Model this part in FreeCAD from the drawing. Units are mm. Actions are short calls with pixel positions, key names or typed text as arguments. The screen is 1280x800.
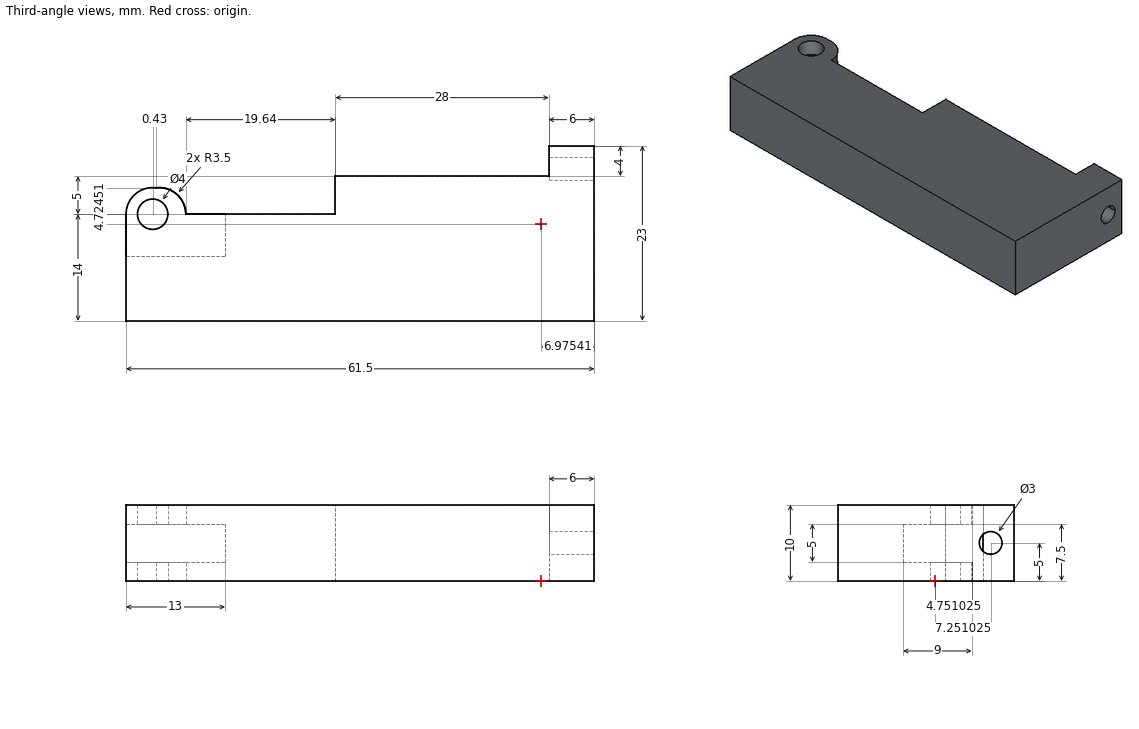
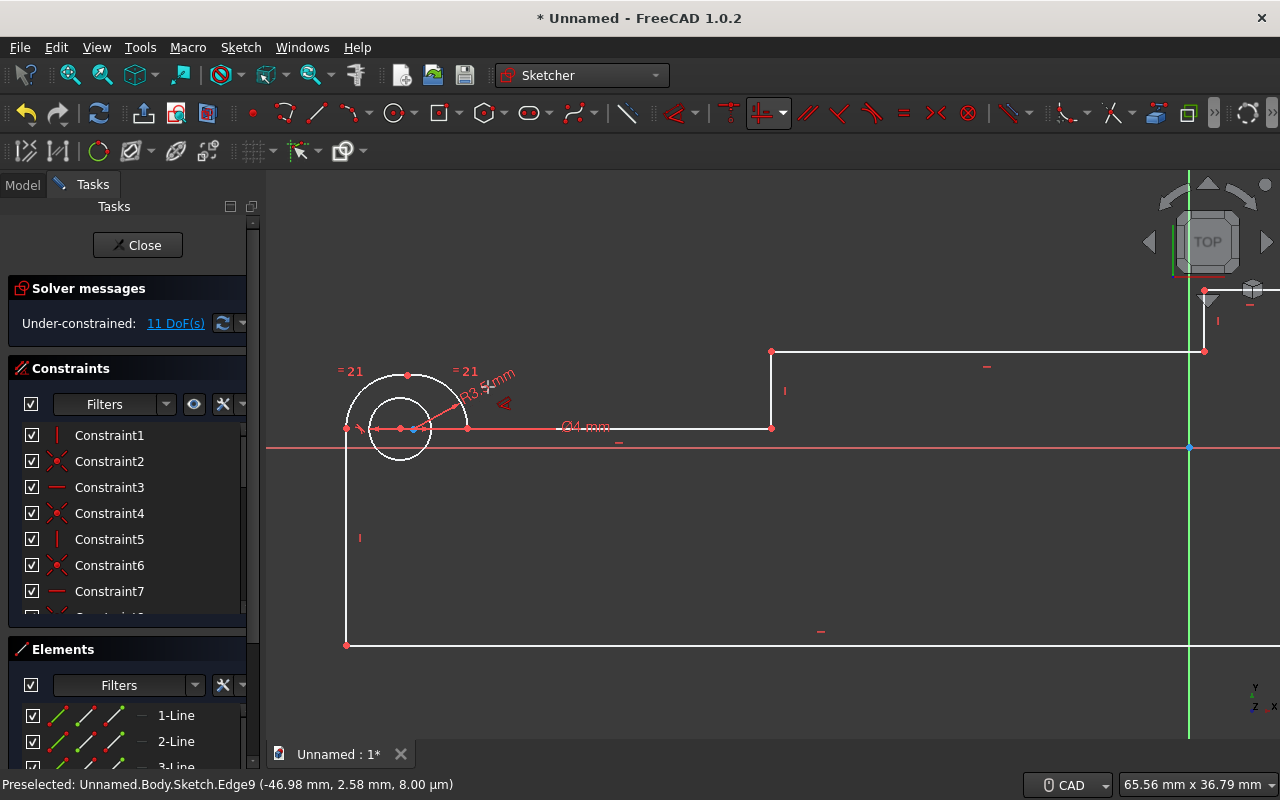
scroll(467, 429, down, 2)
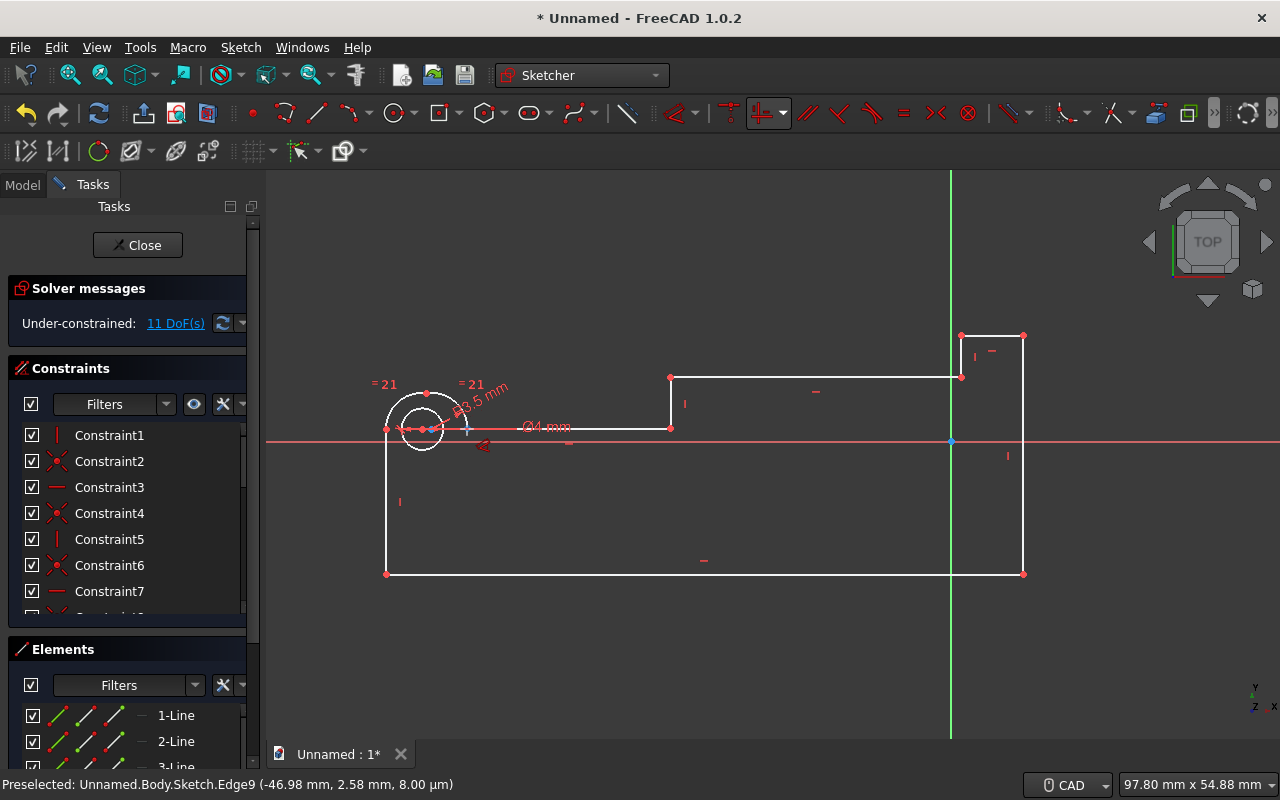
click(1004, 336)
click(992, 302)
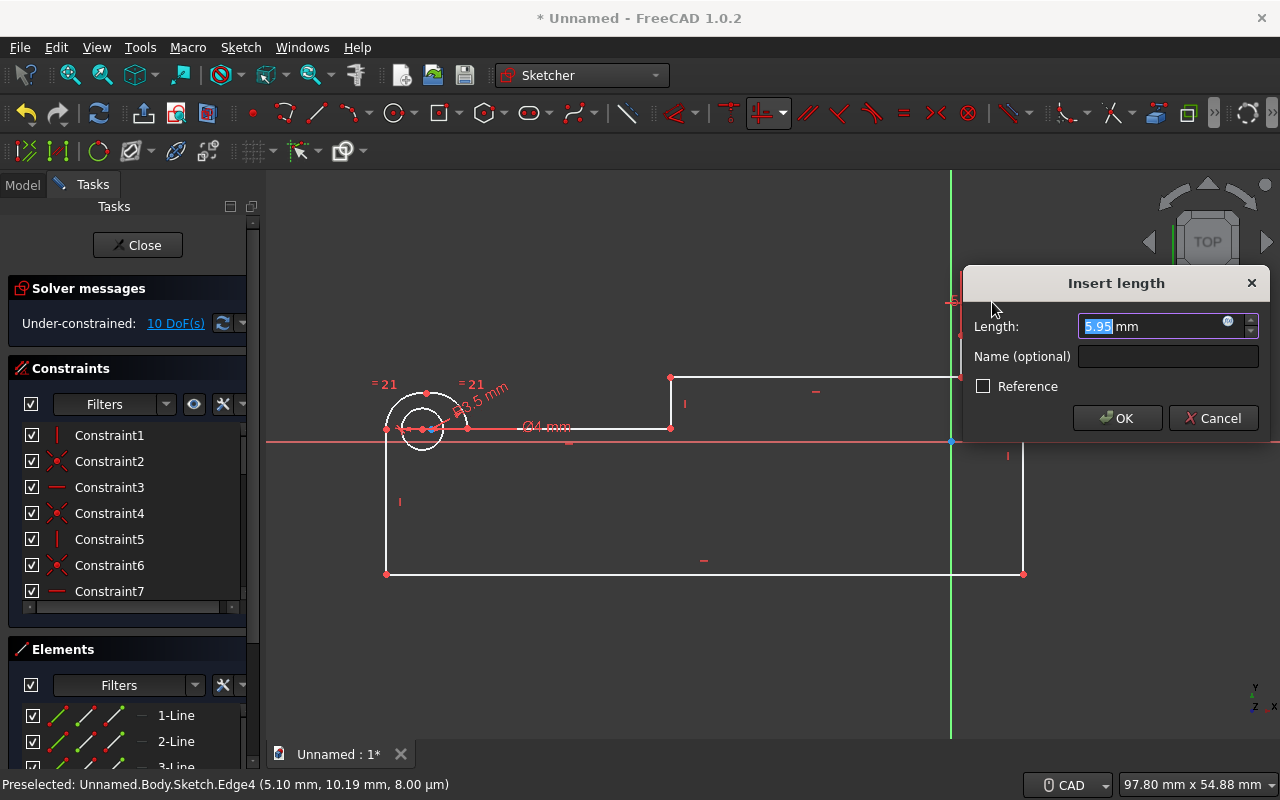
text(6)
key(Return)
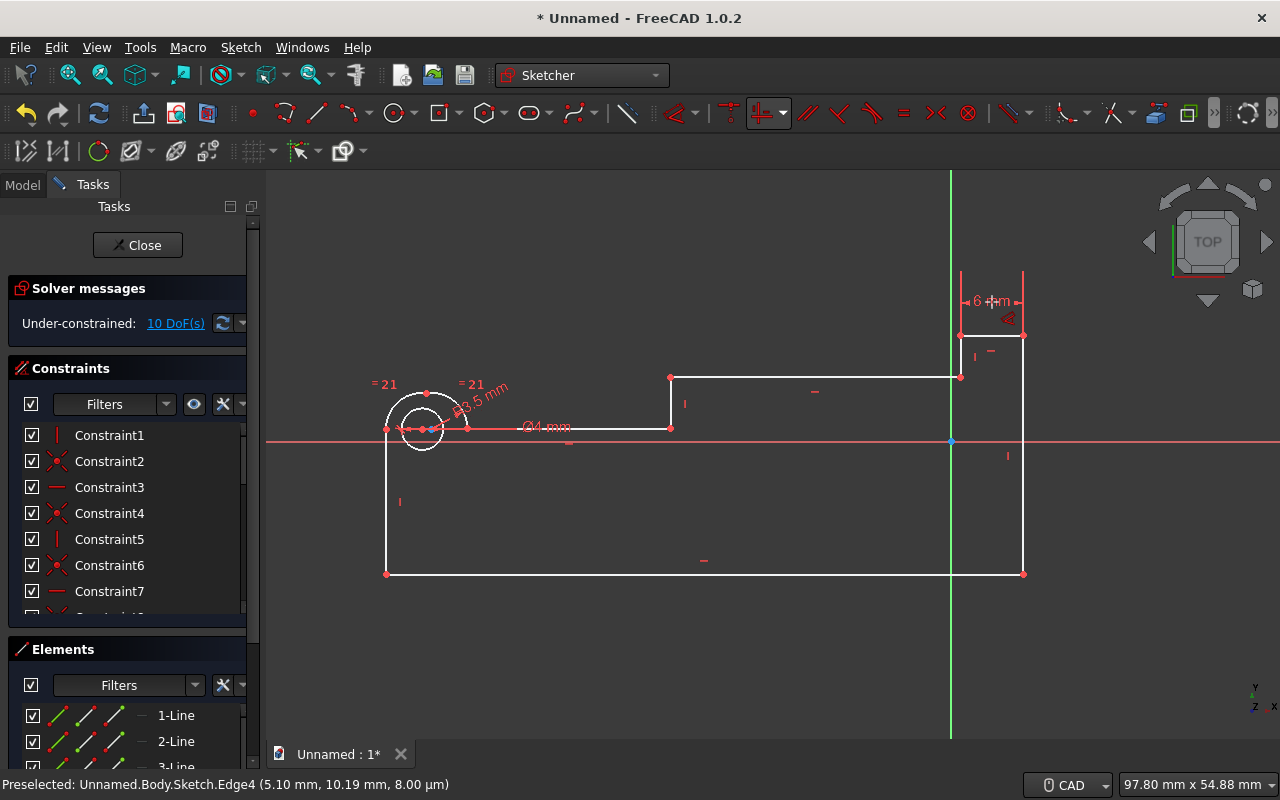
scroll(961, 348, up, 2)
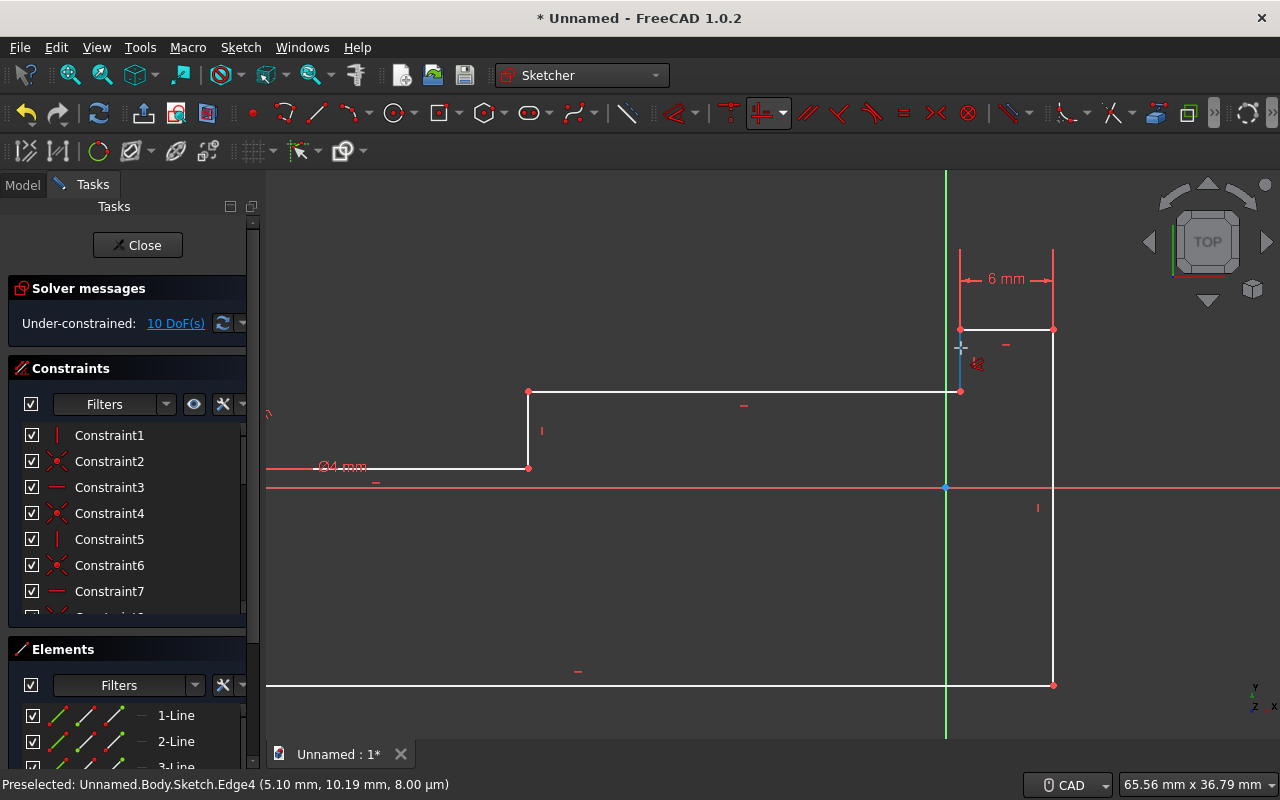
click(960, 348)
click(994, 361)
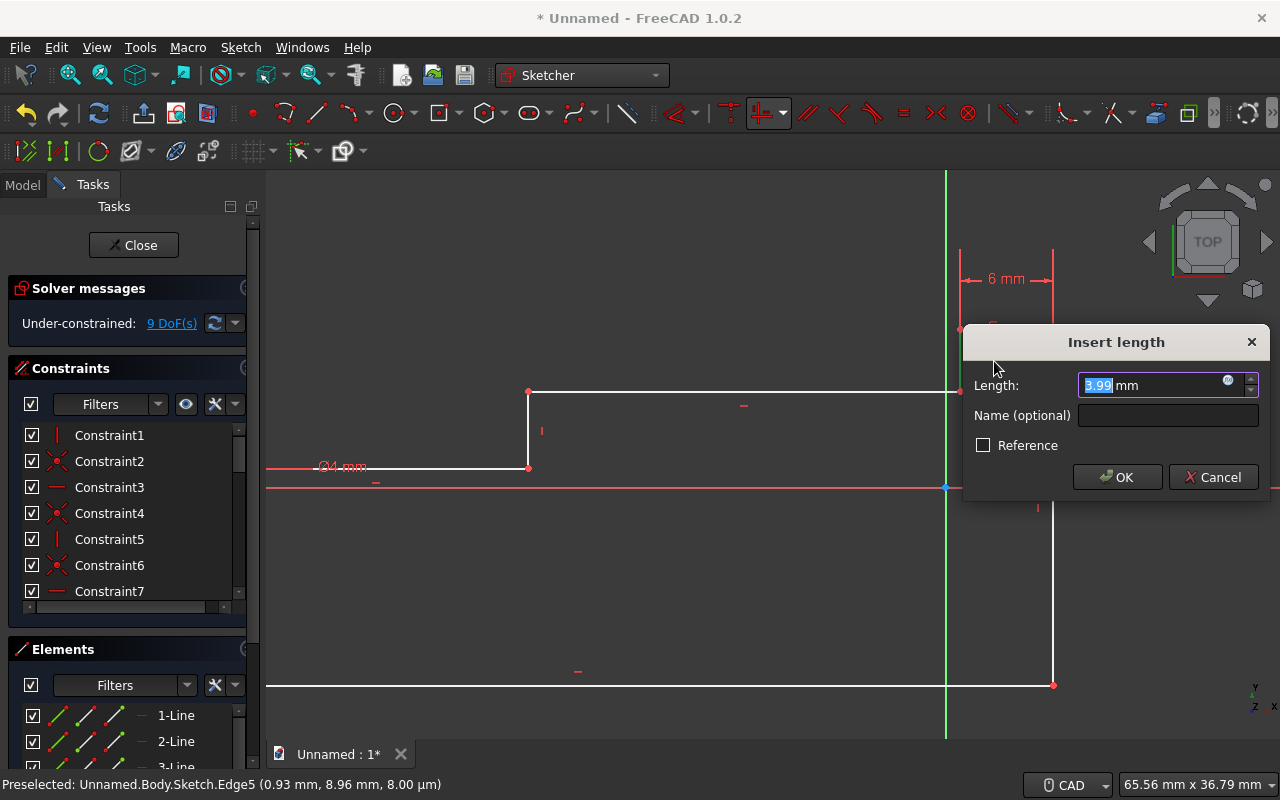
text(4)
key(Return)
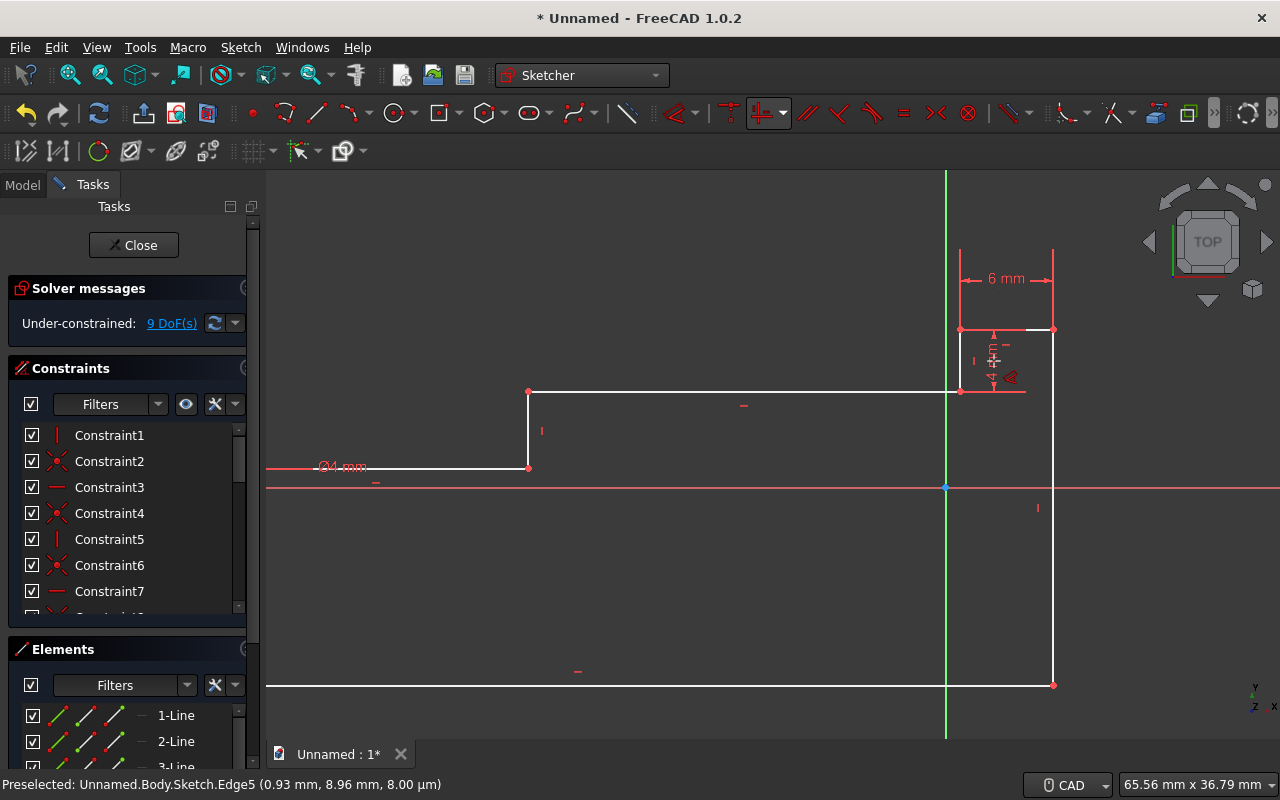
click(528, 415)
click(494, 430)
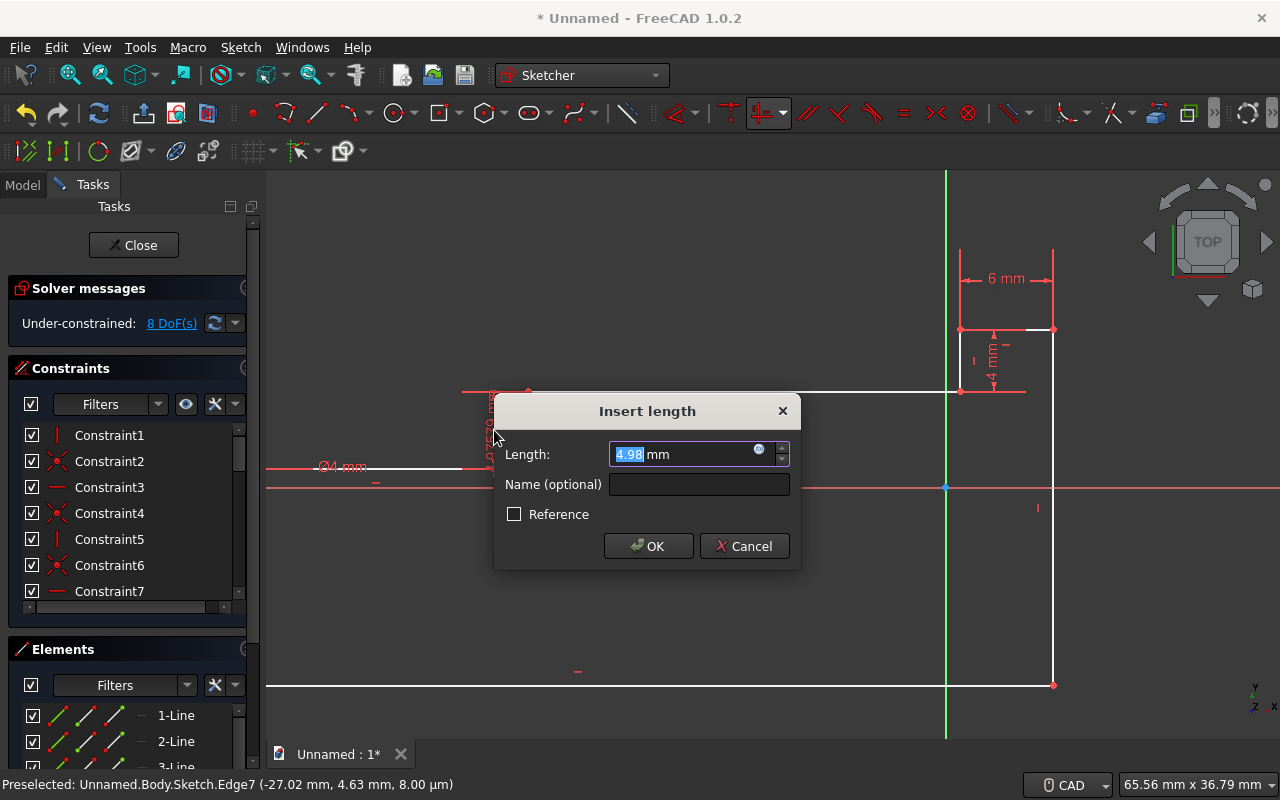
text(5)
key(Return)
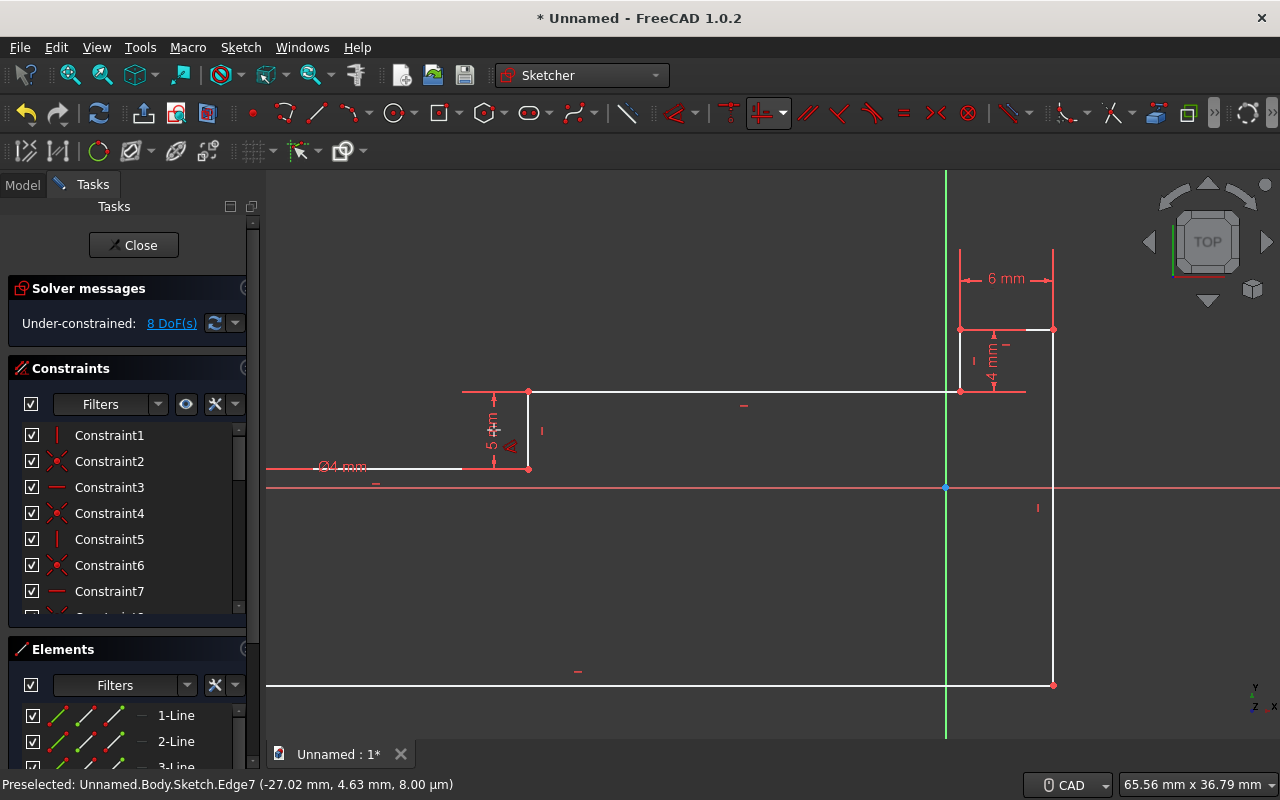
scroll(961, 348, down, 2)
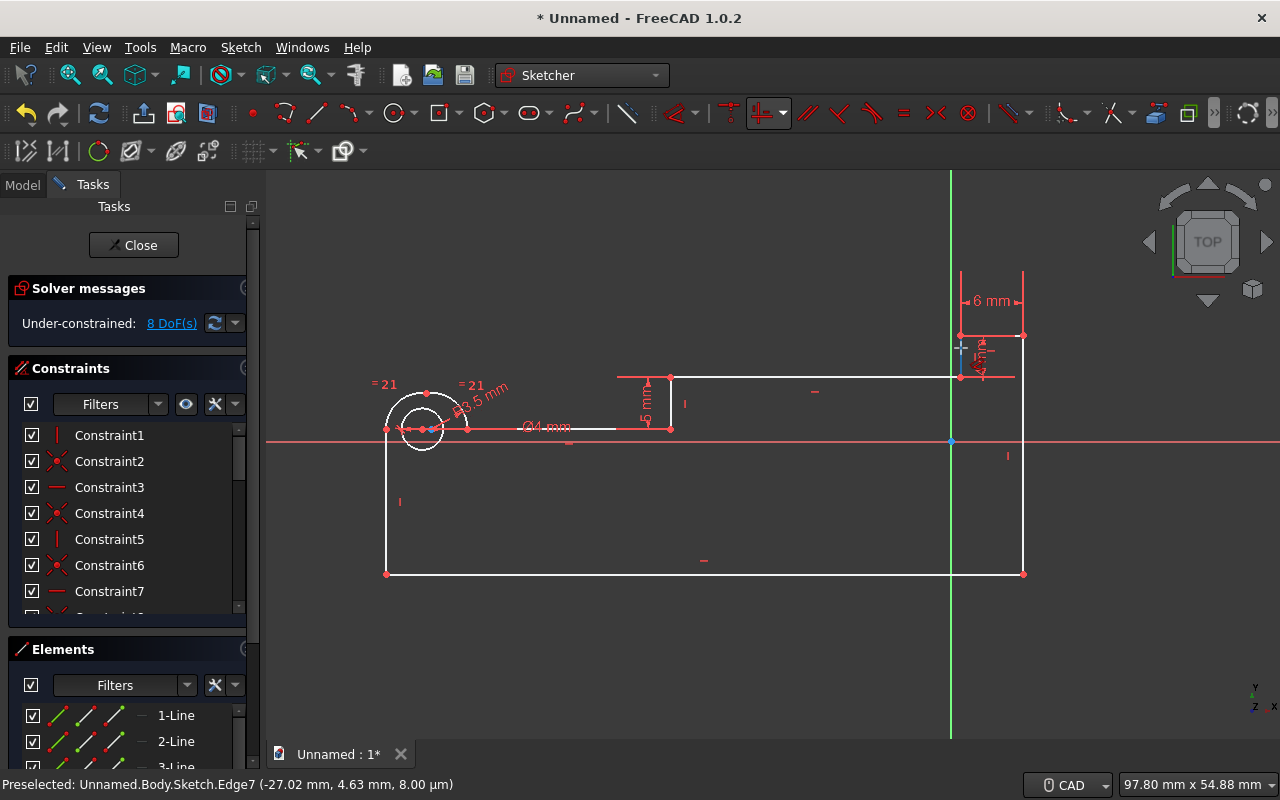
click(386, 473)
click(352, 502)